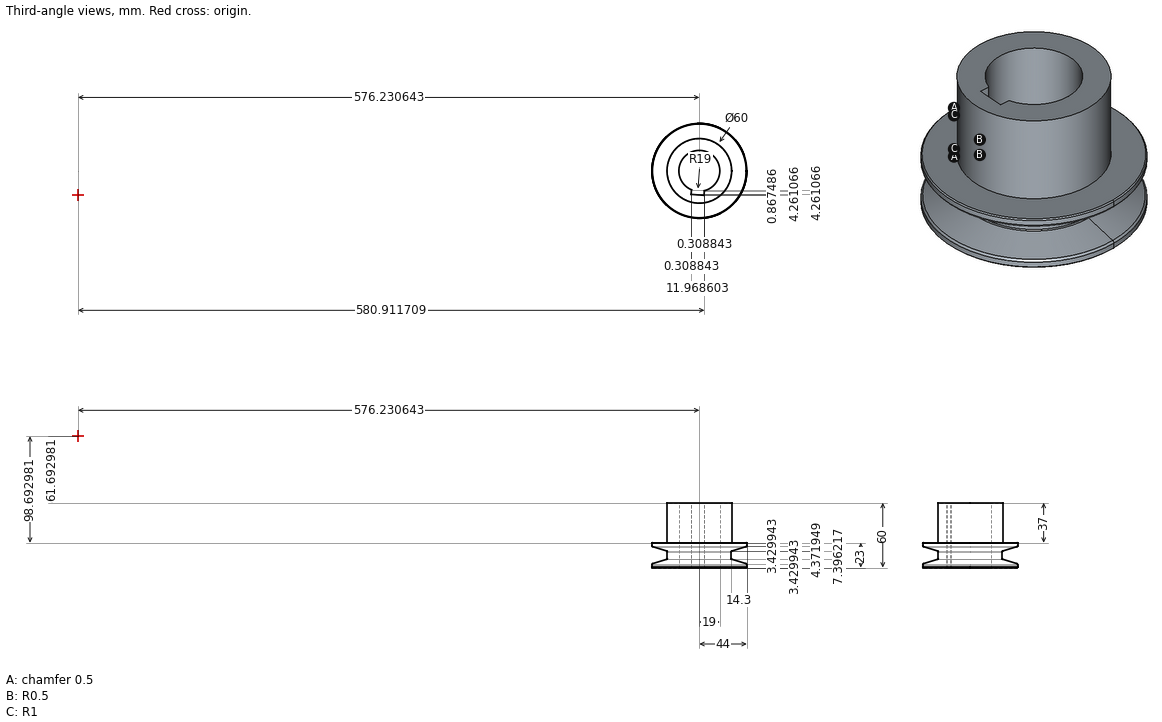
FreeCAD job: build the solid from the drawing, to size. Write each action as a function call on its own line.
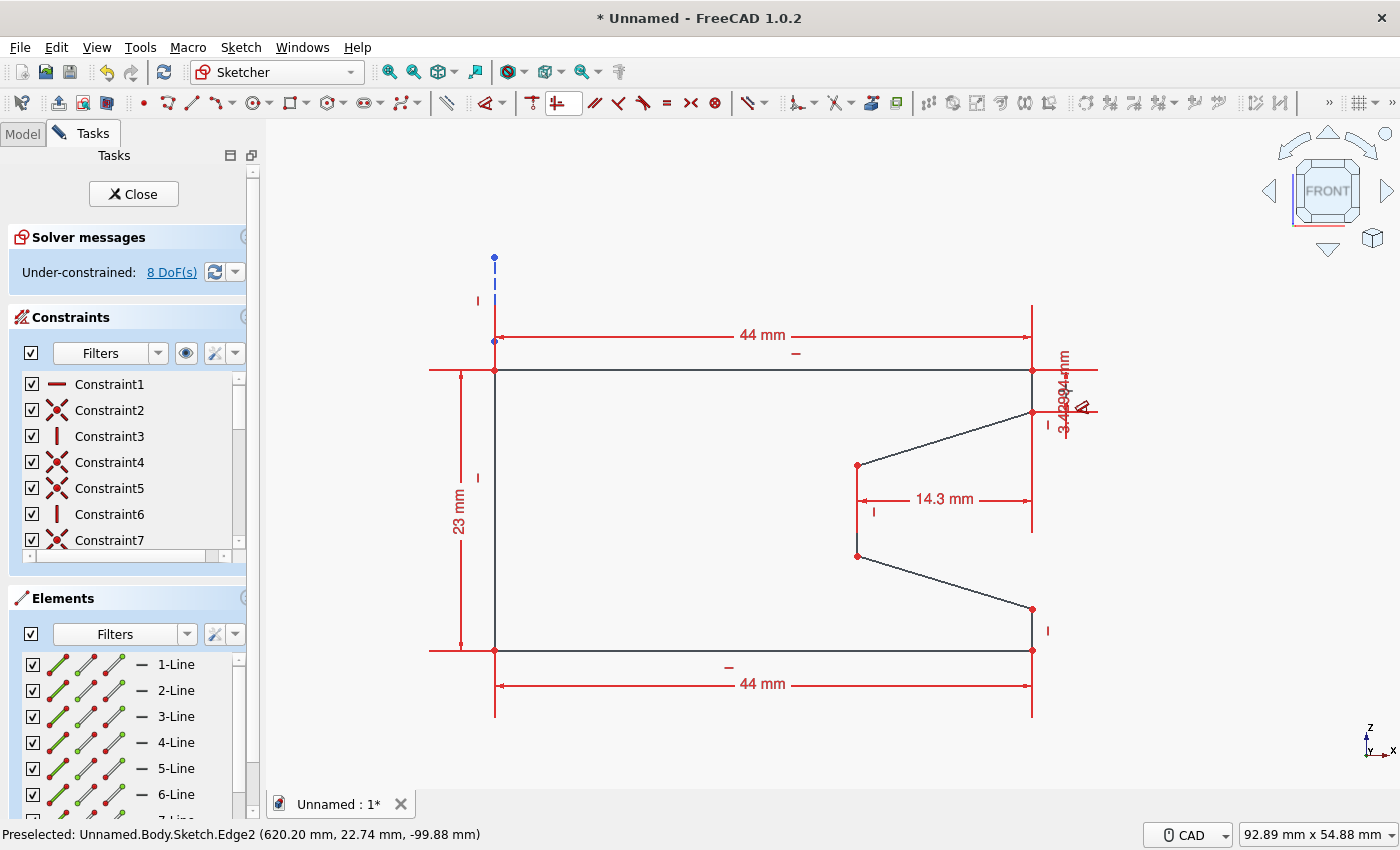
click(857, 493)
click(891, 532)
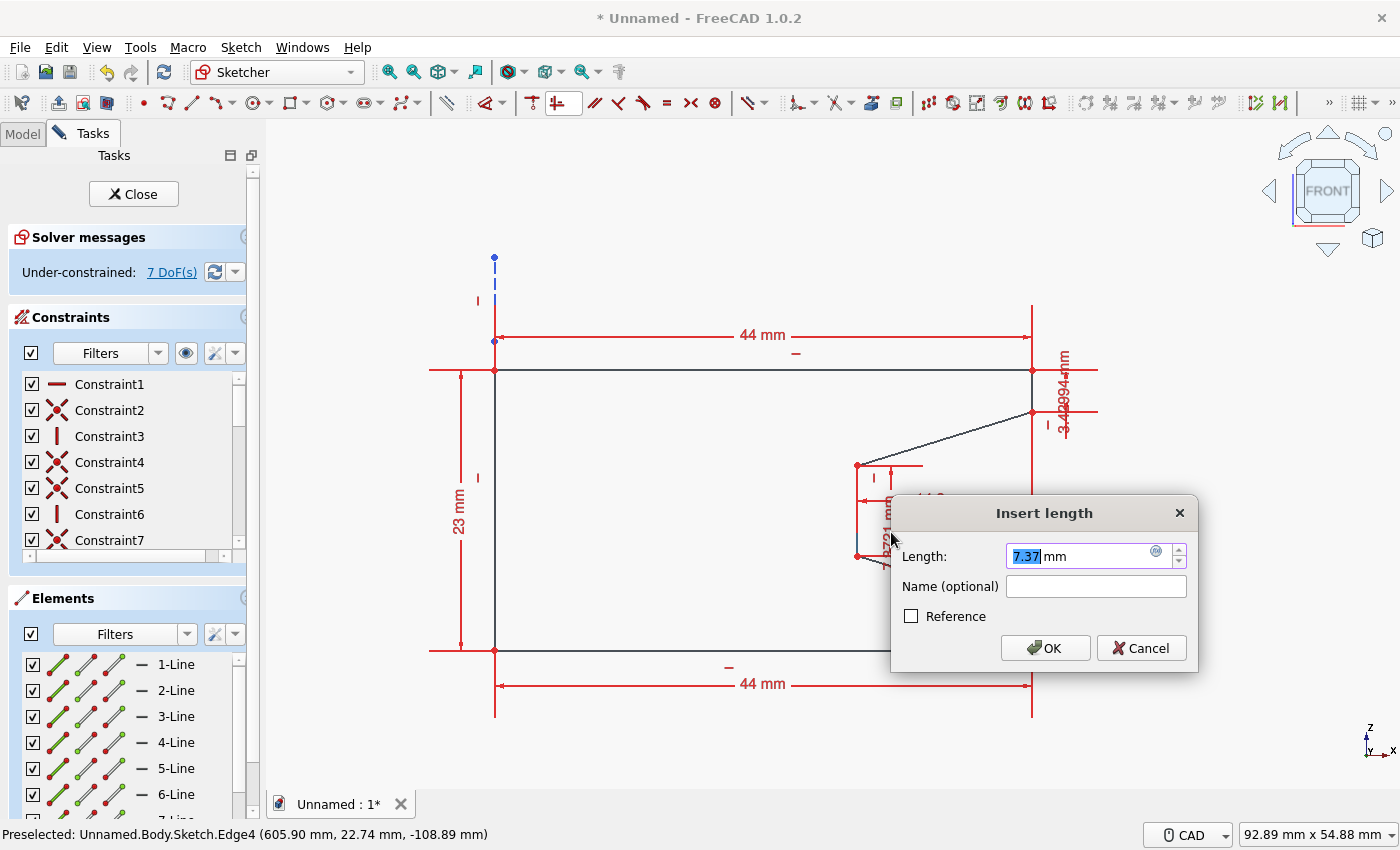
text(7.396217)
key(Return)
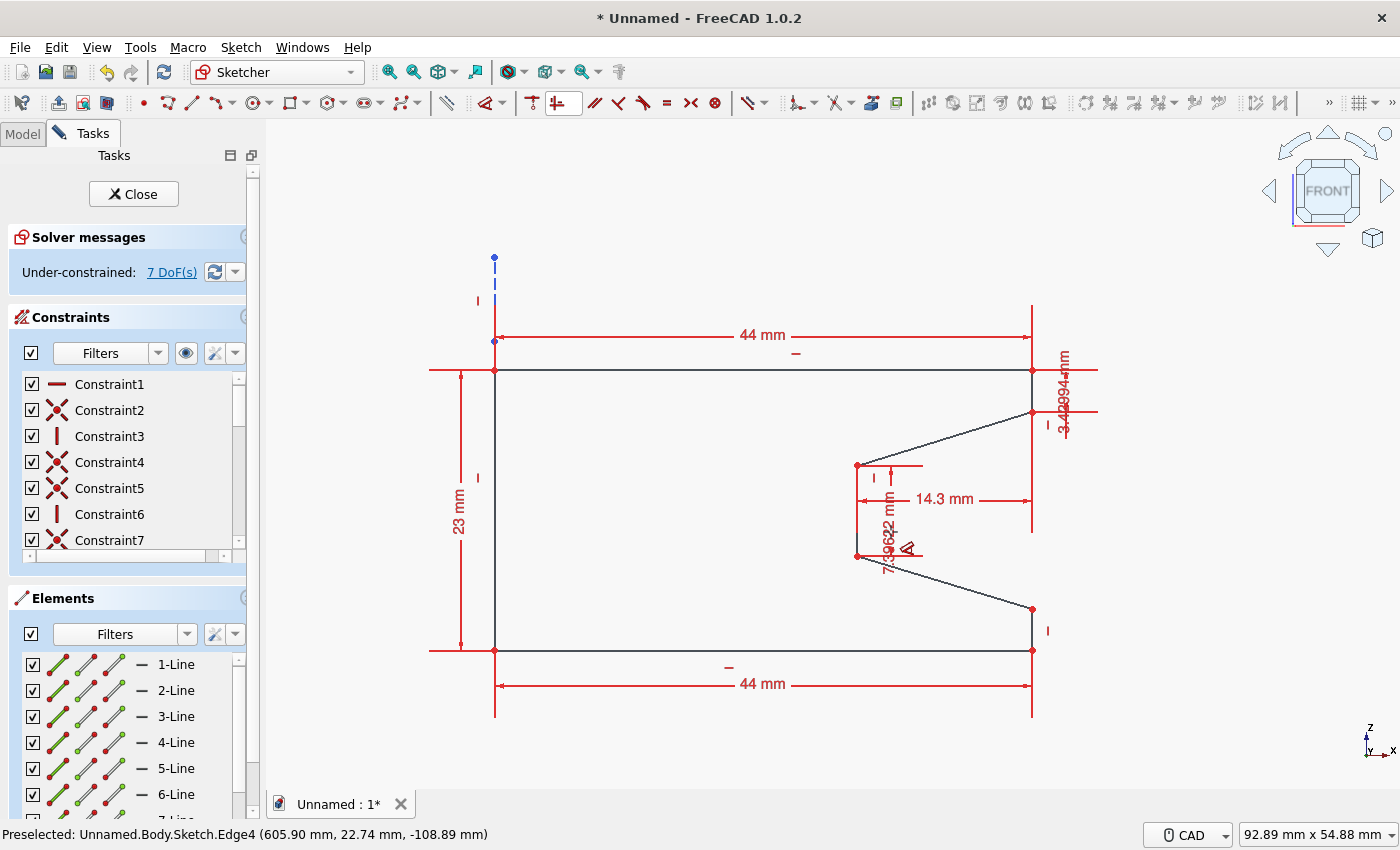
click(1032, 622)
click(1066, 630)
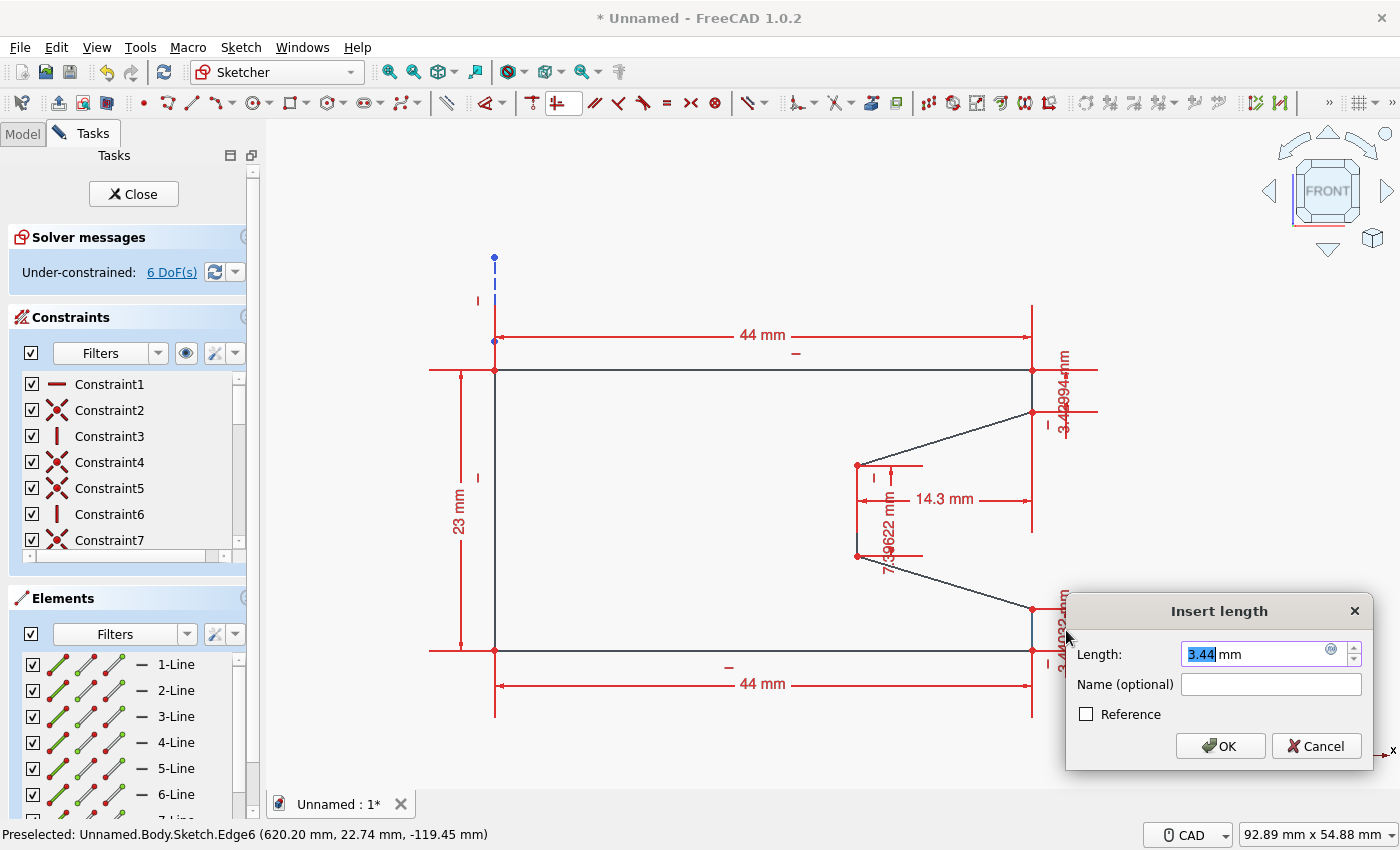
text(3.429943)
key(Return)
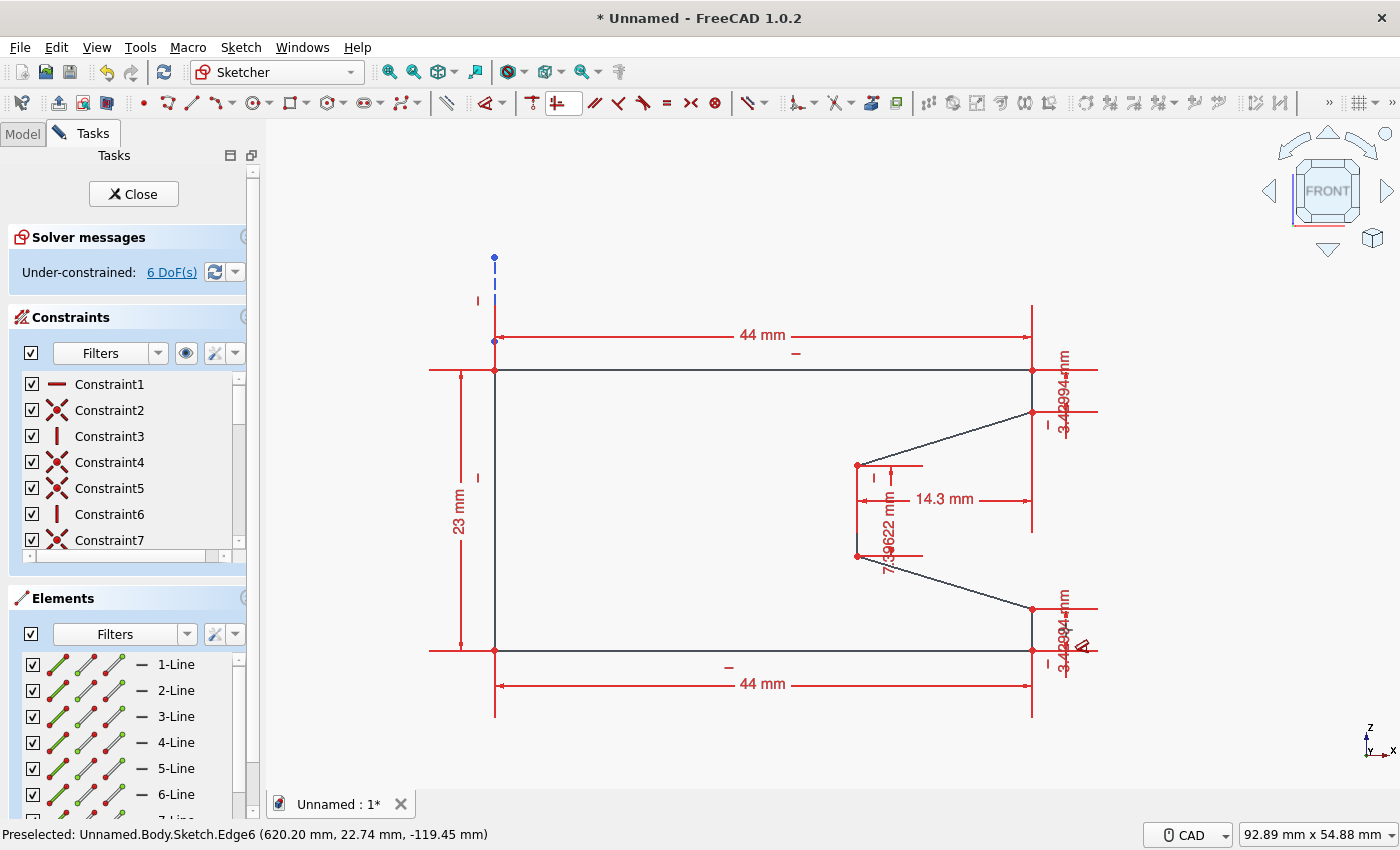
click(980, 428)
click(1066, 439)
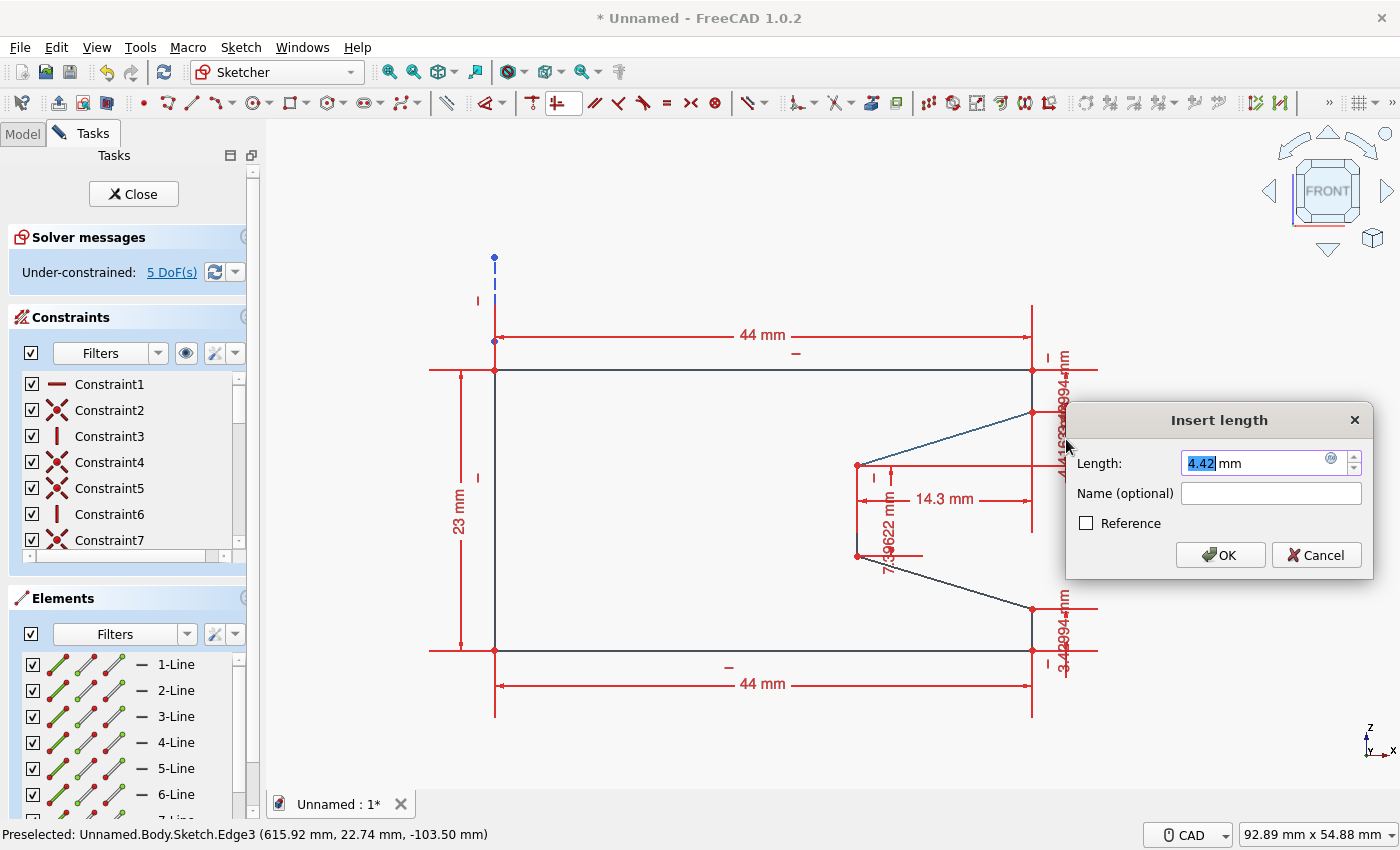
text(4.371949)
key(Return)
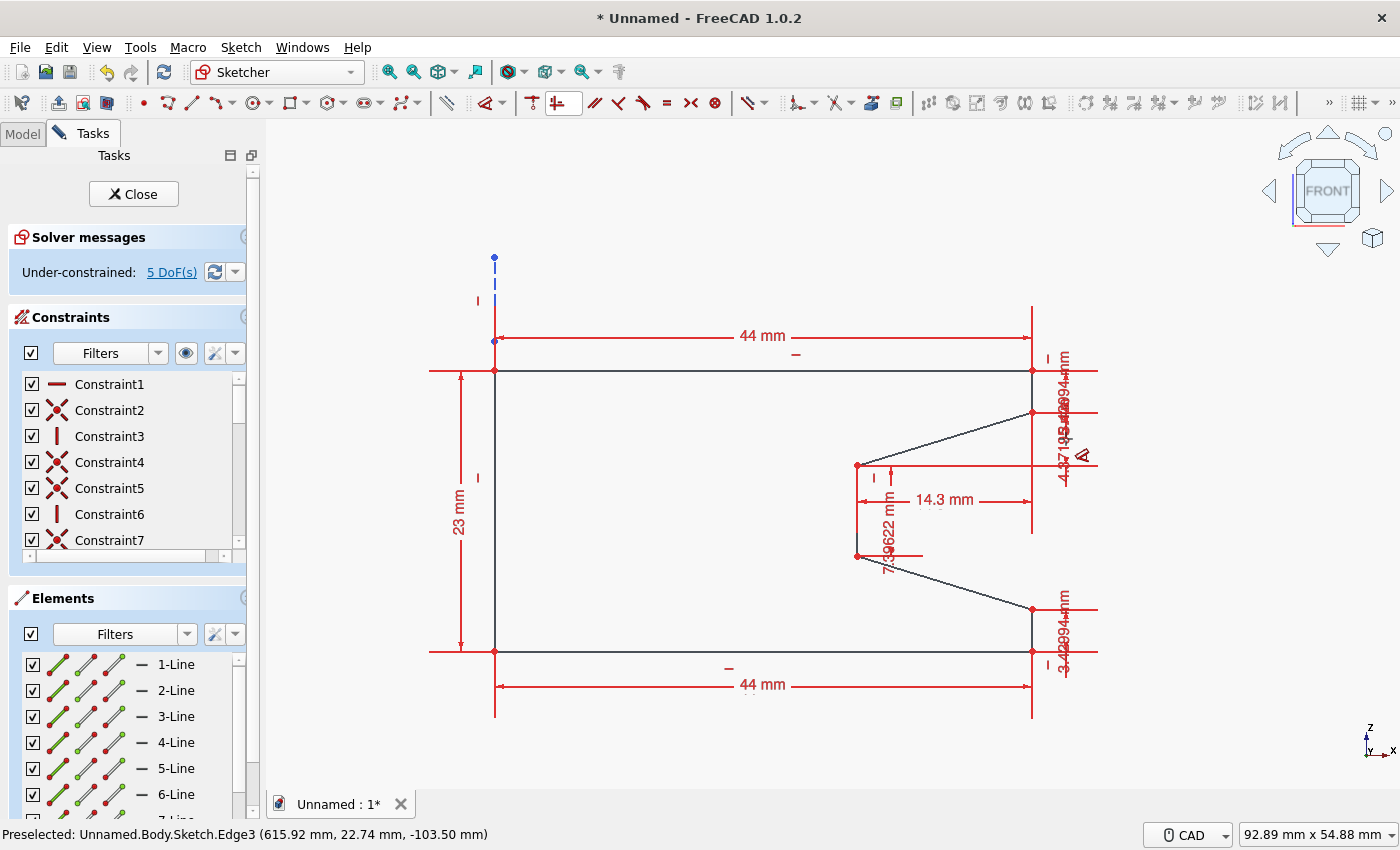
click(495, 371)
click(529, 259)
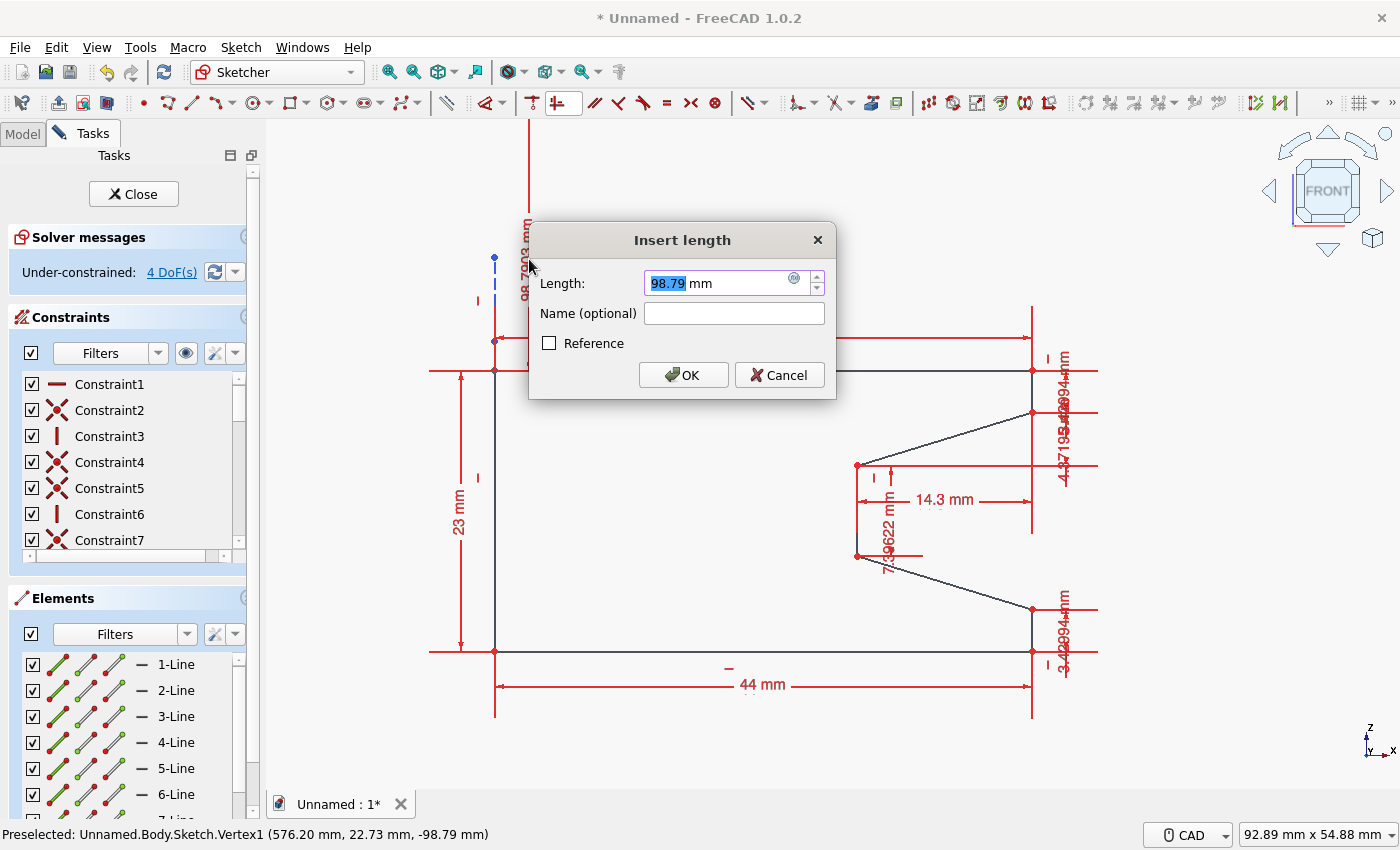
text(98.692981)
key(Return)